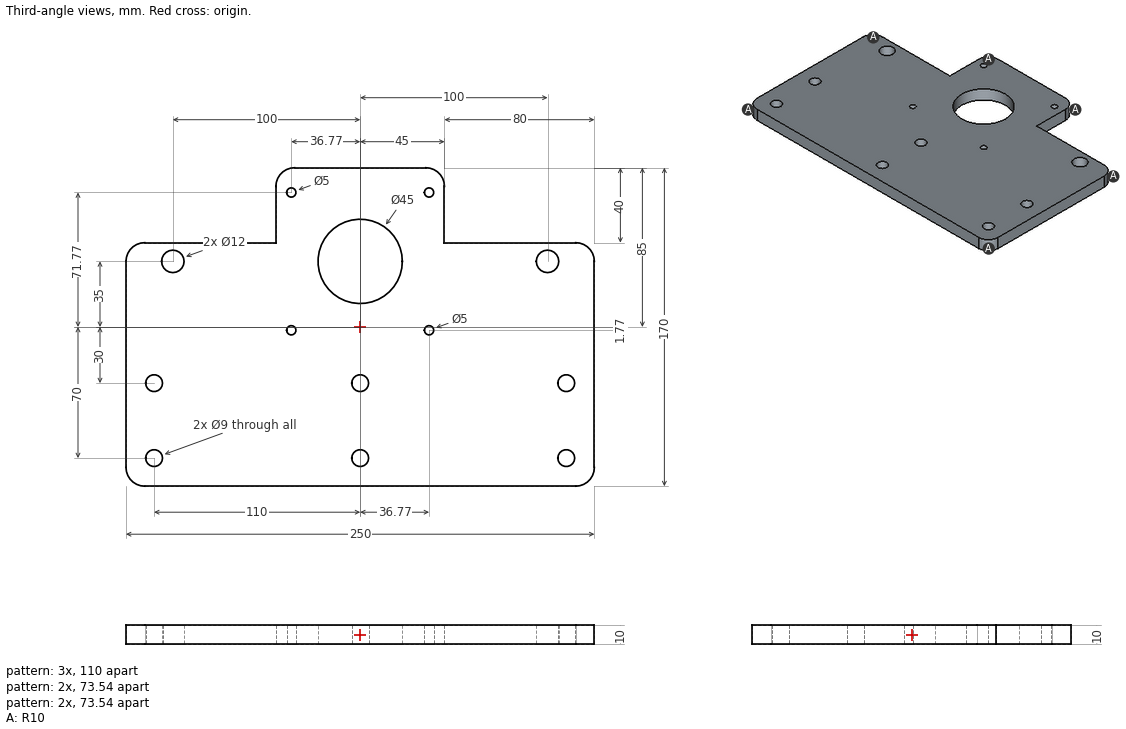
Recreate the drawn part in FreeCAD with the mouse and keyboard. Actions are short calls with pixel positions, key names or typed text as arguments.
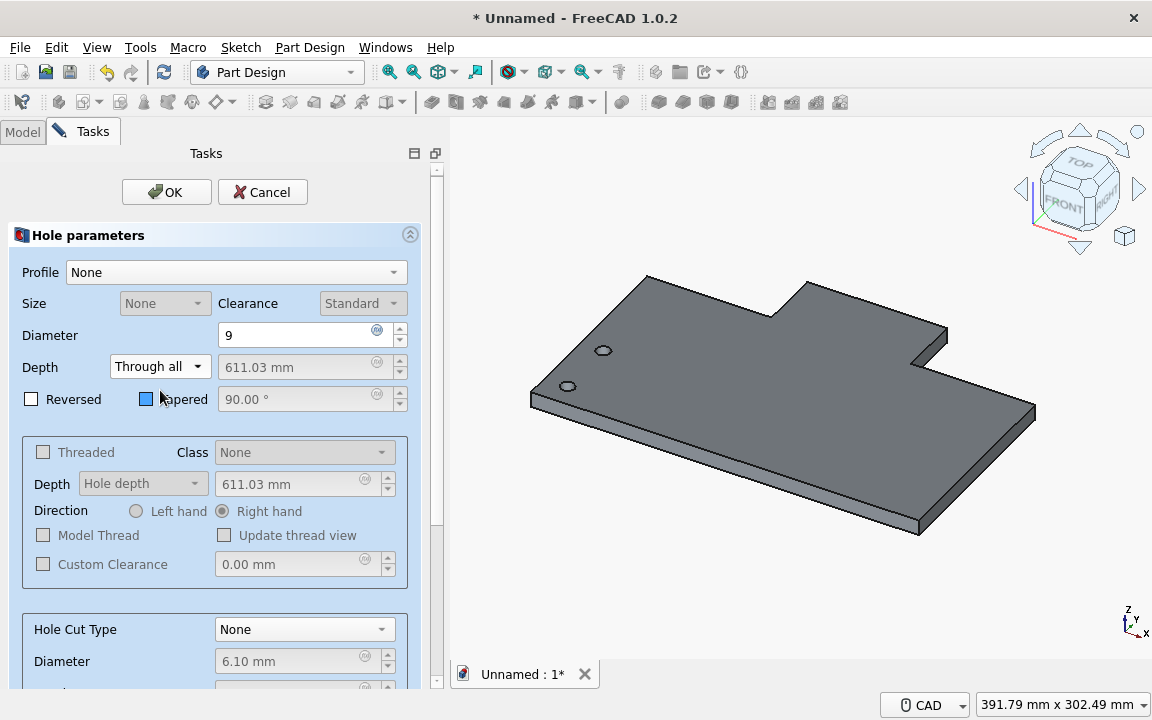
click(167, 192)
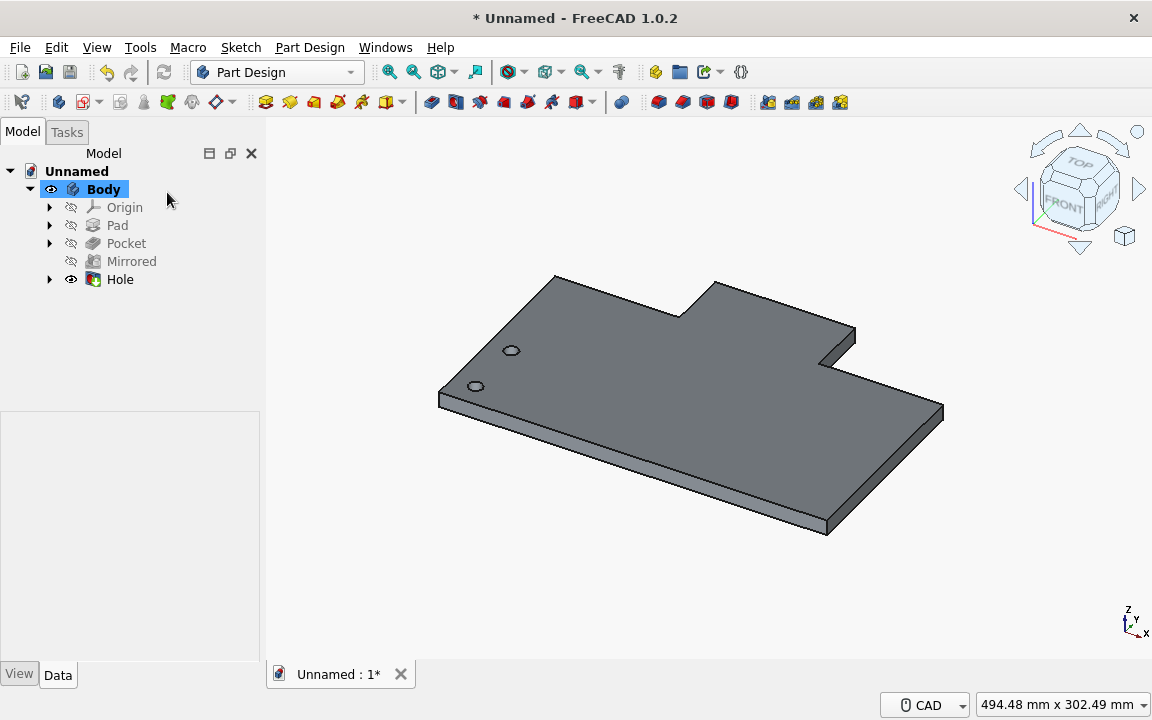
click(116, 279)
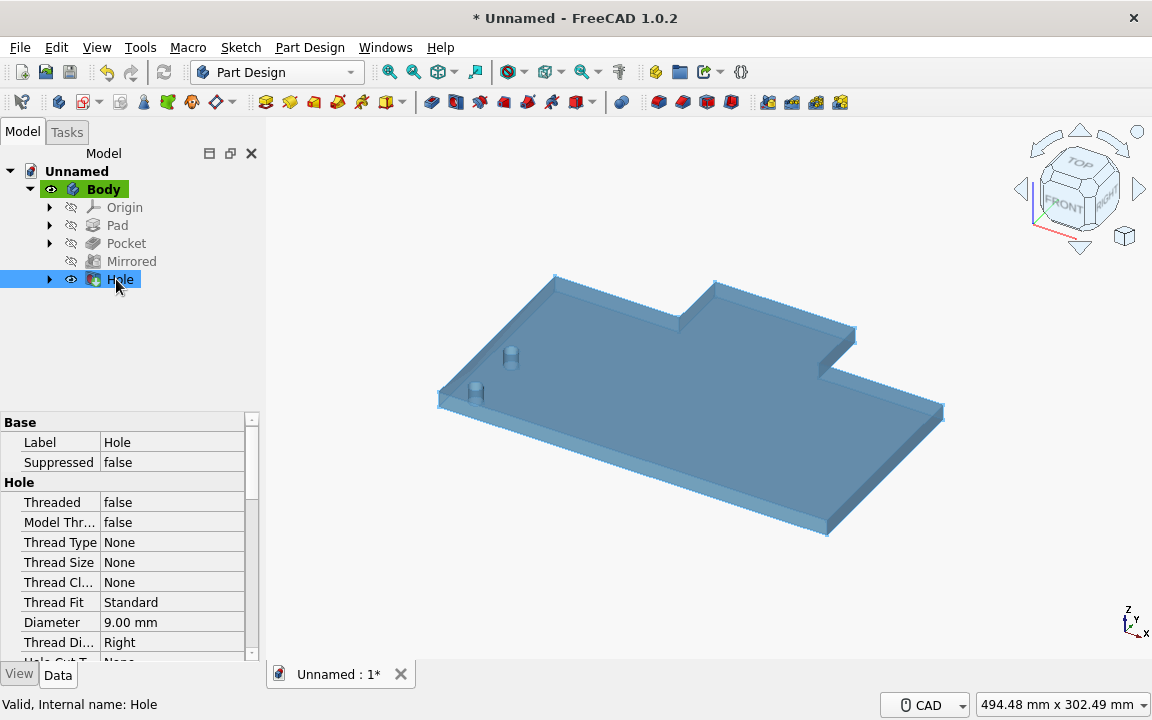
click(792, 102)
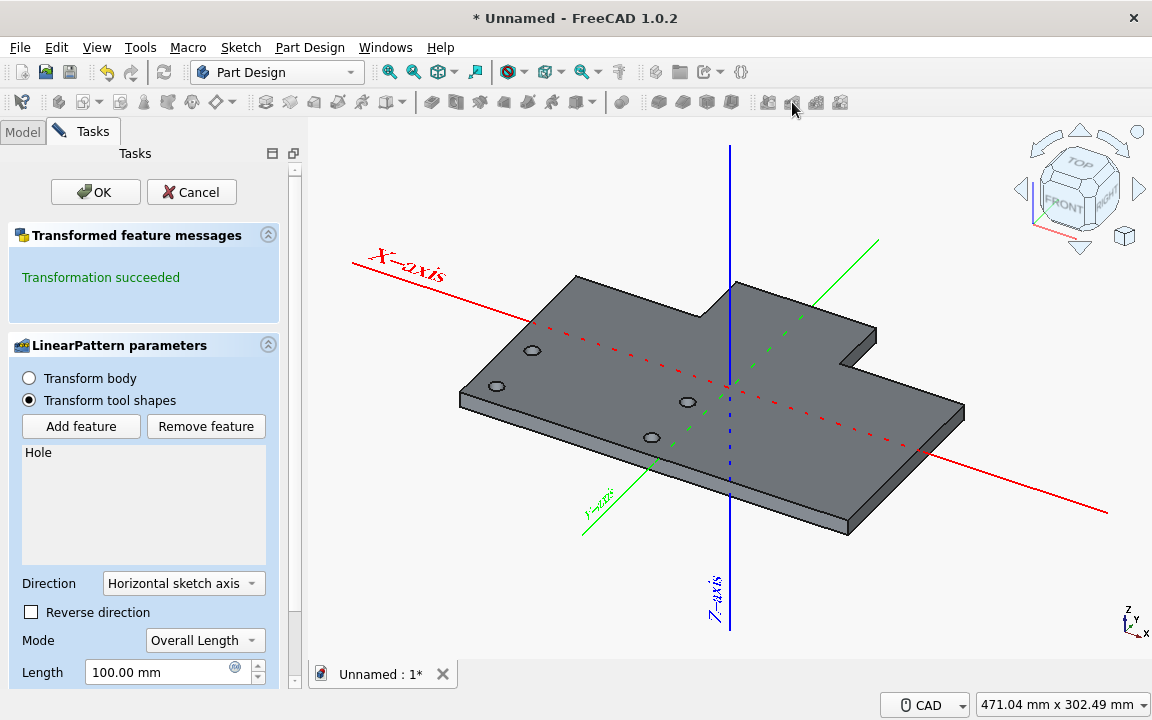
click(184, 584)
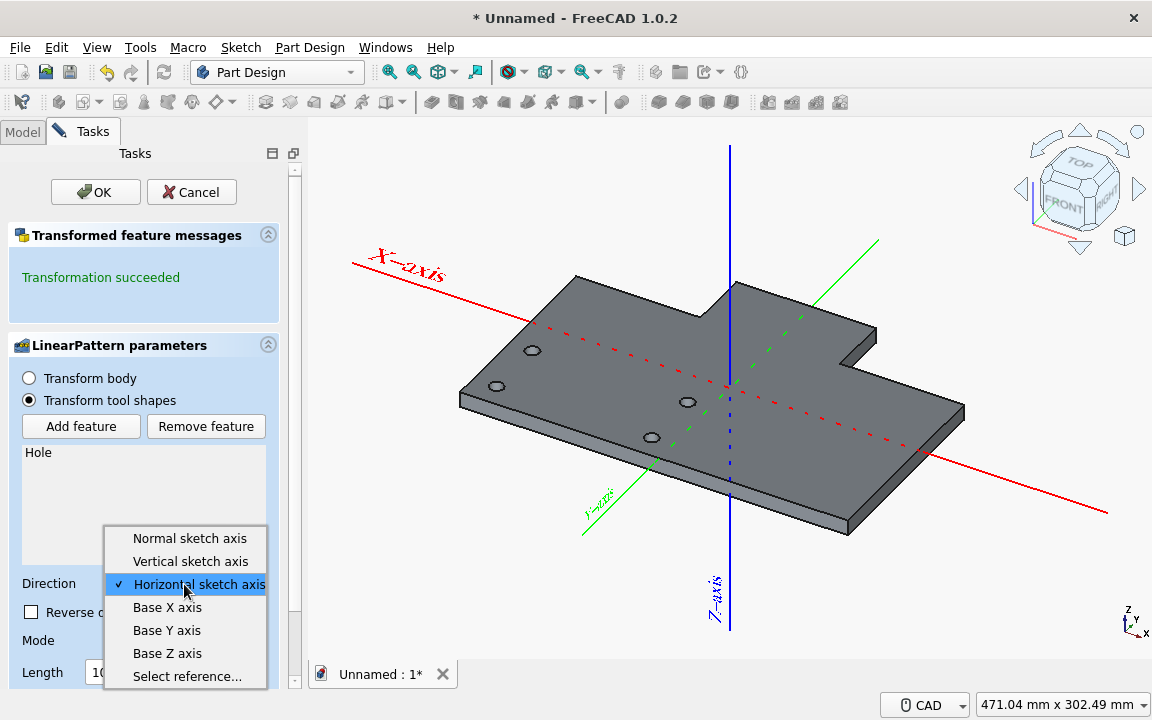
click(184, 608)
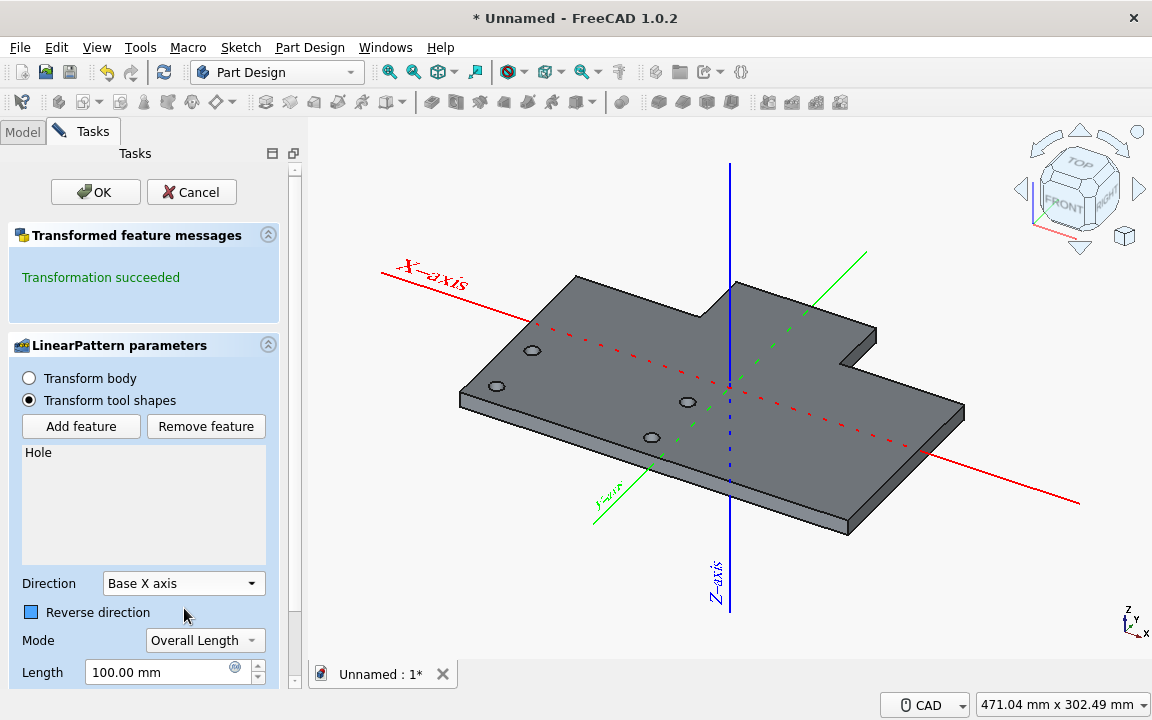
click(206, 640)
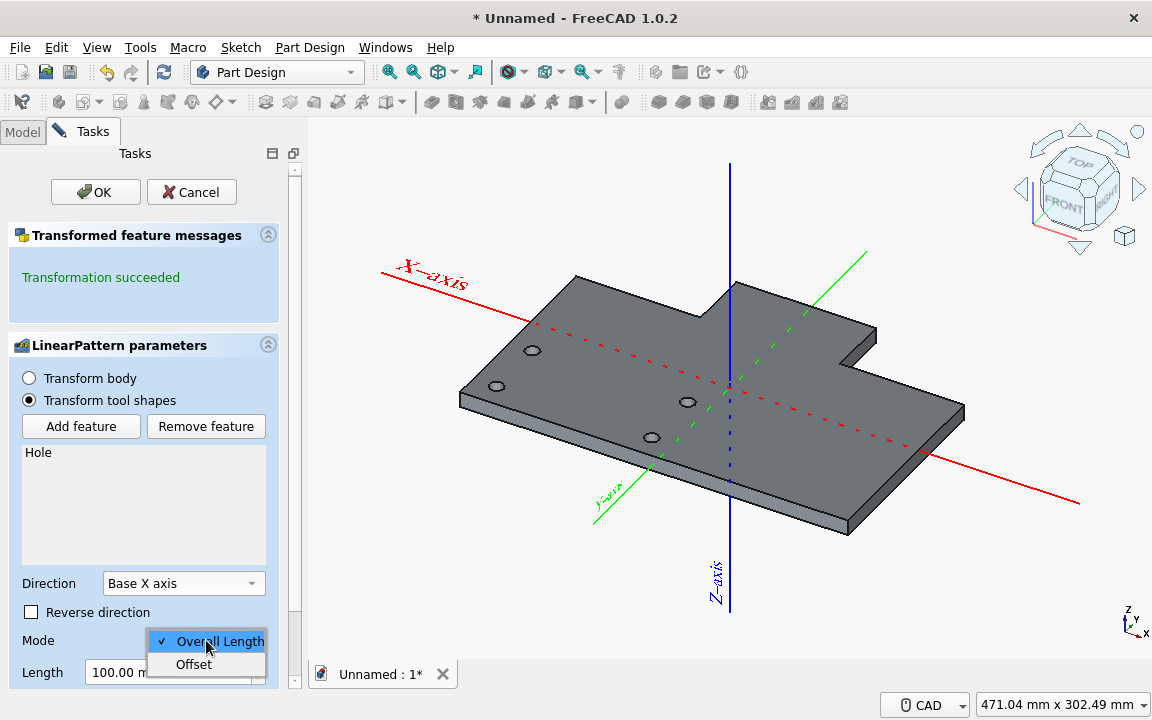
click(206, 664)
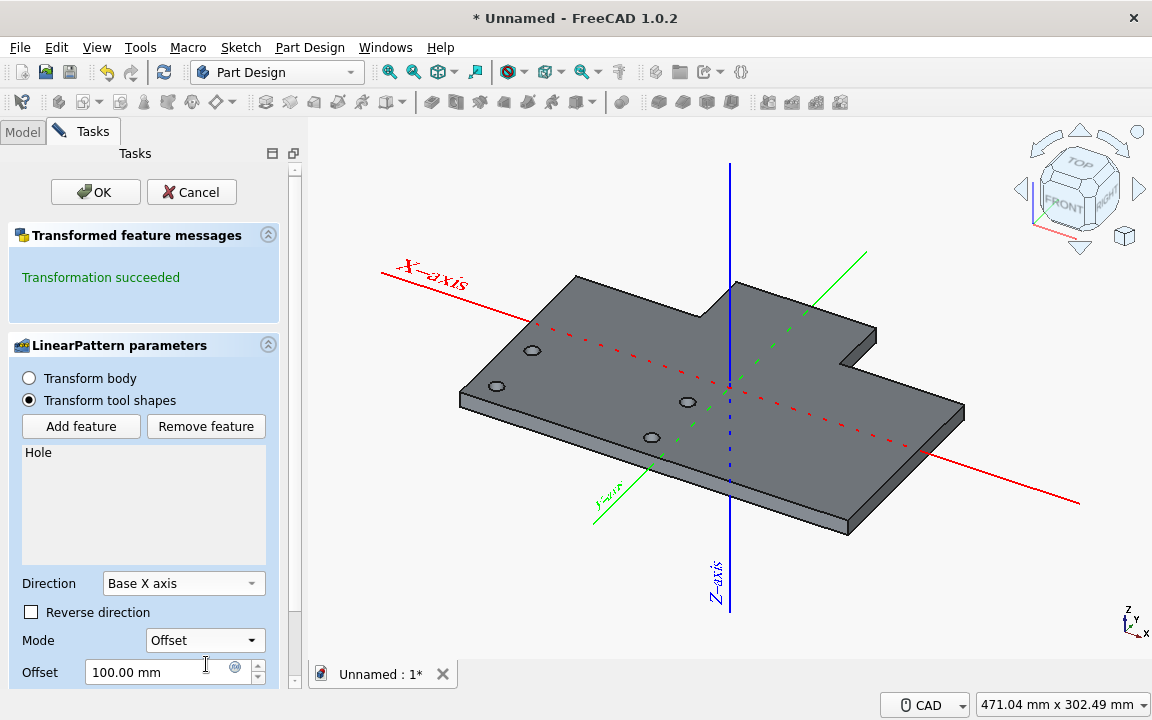
triple_click(168, 672)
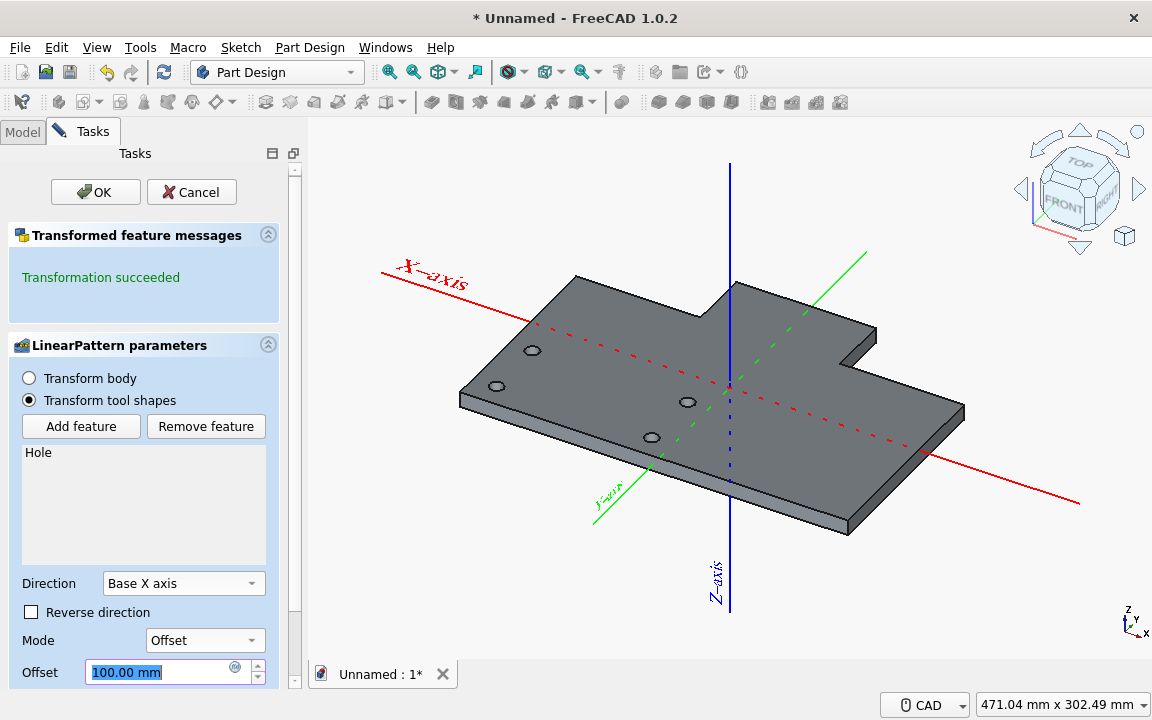
text(110)
key(Tab)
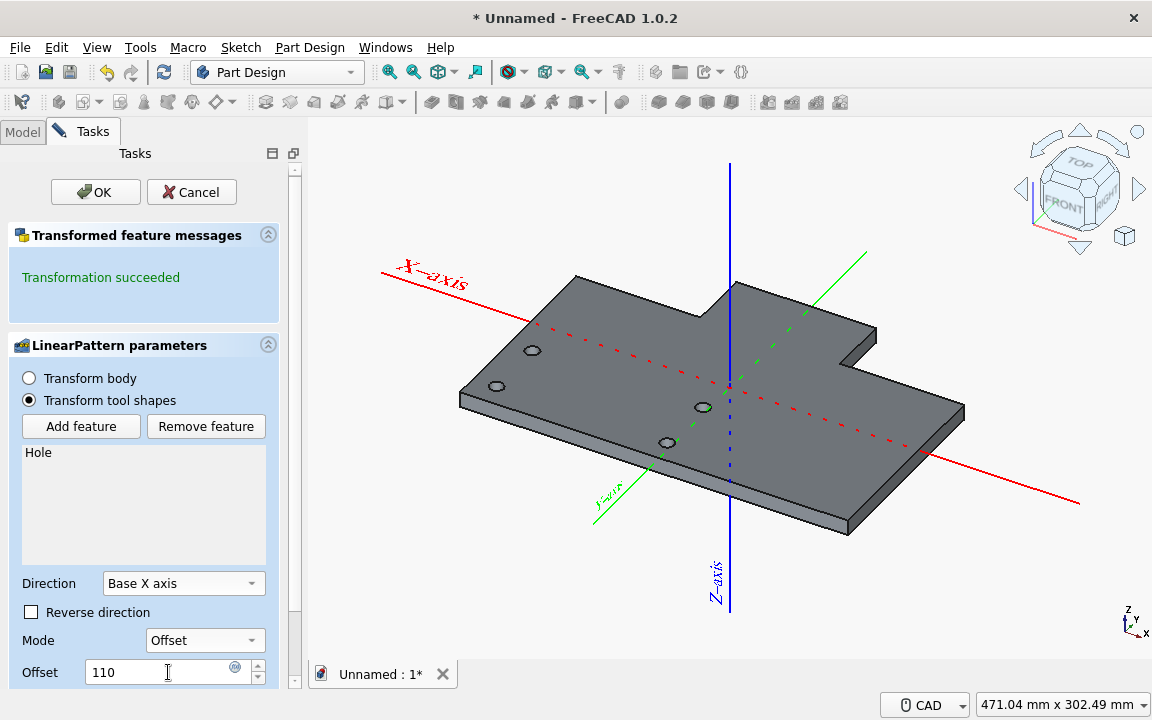
scroll(295, 426, down, 2)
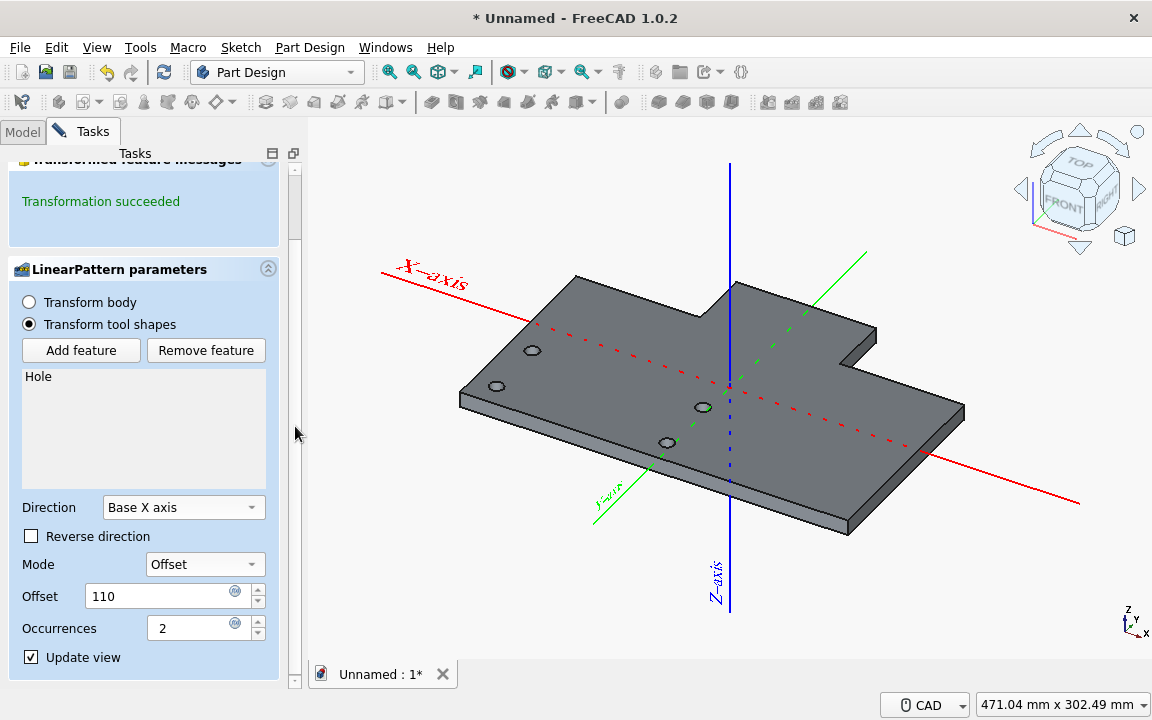
triple_click(198, 628)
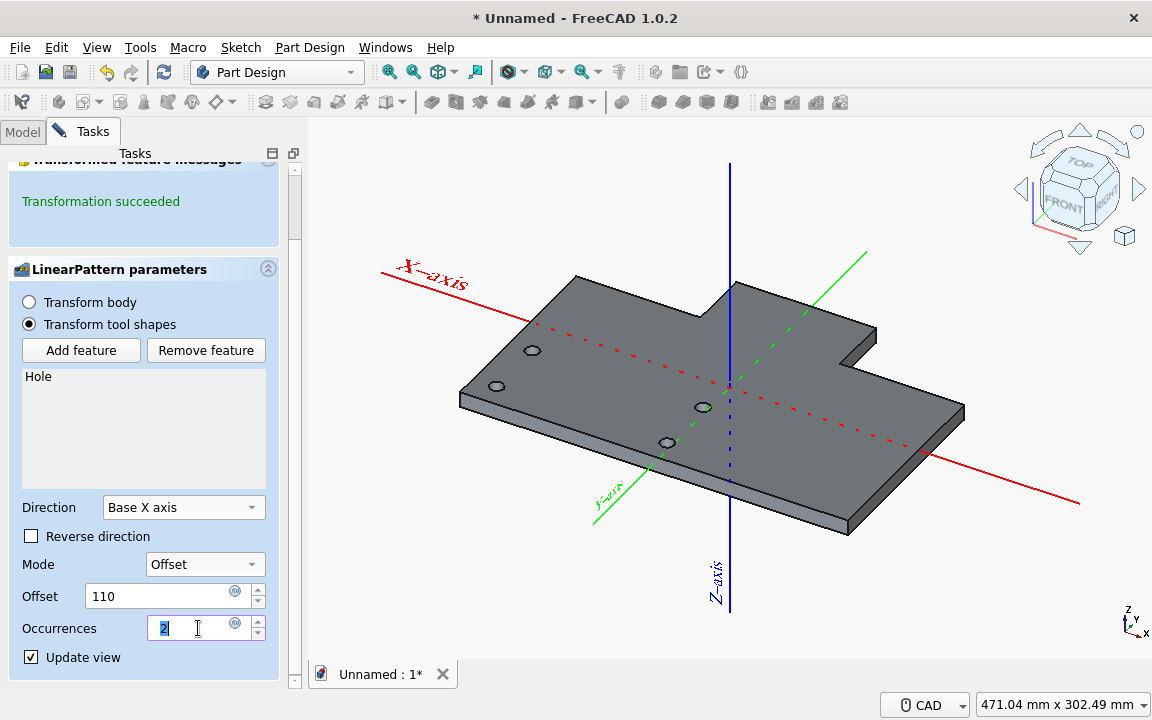
text(3)
key(Tab)